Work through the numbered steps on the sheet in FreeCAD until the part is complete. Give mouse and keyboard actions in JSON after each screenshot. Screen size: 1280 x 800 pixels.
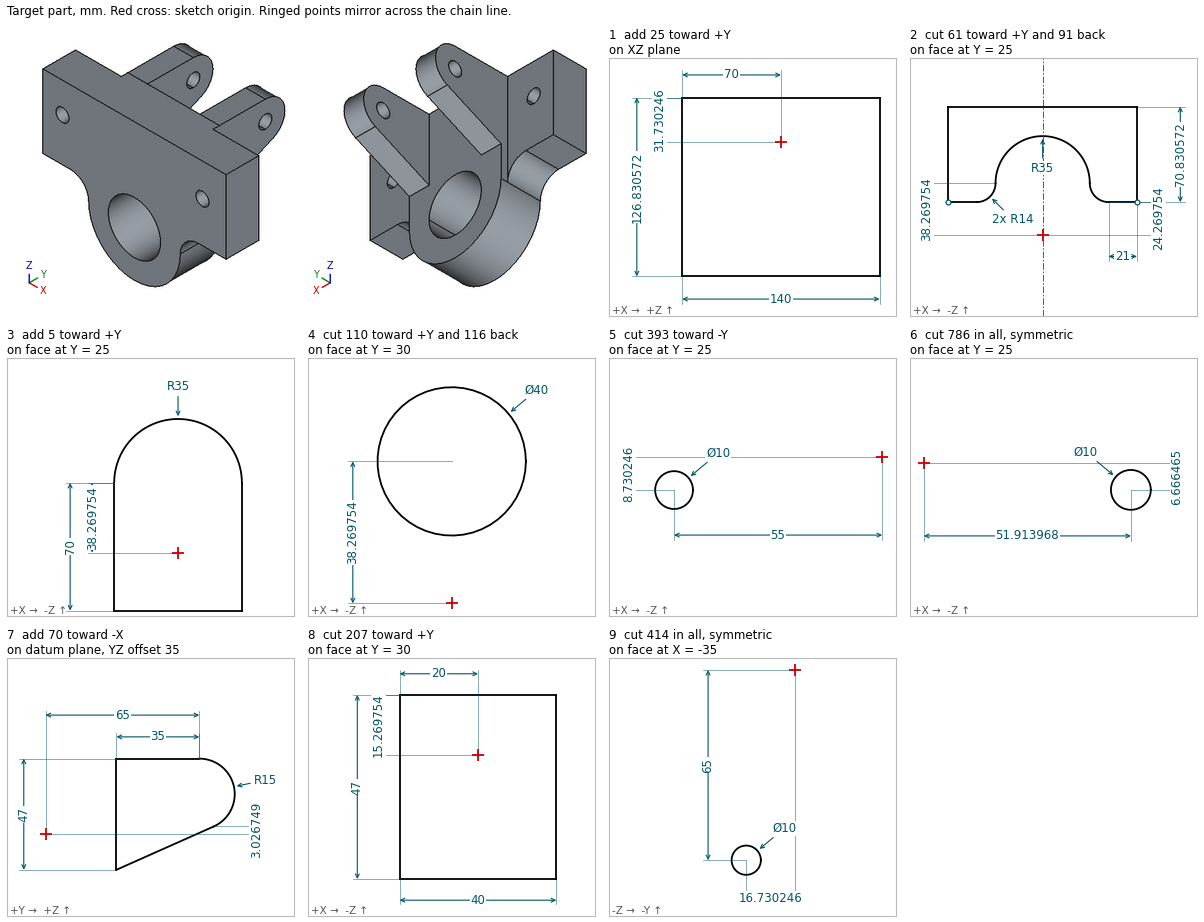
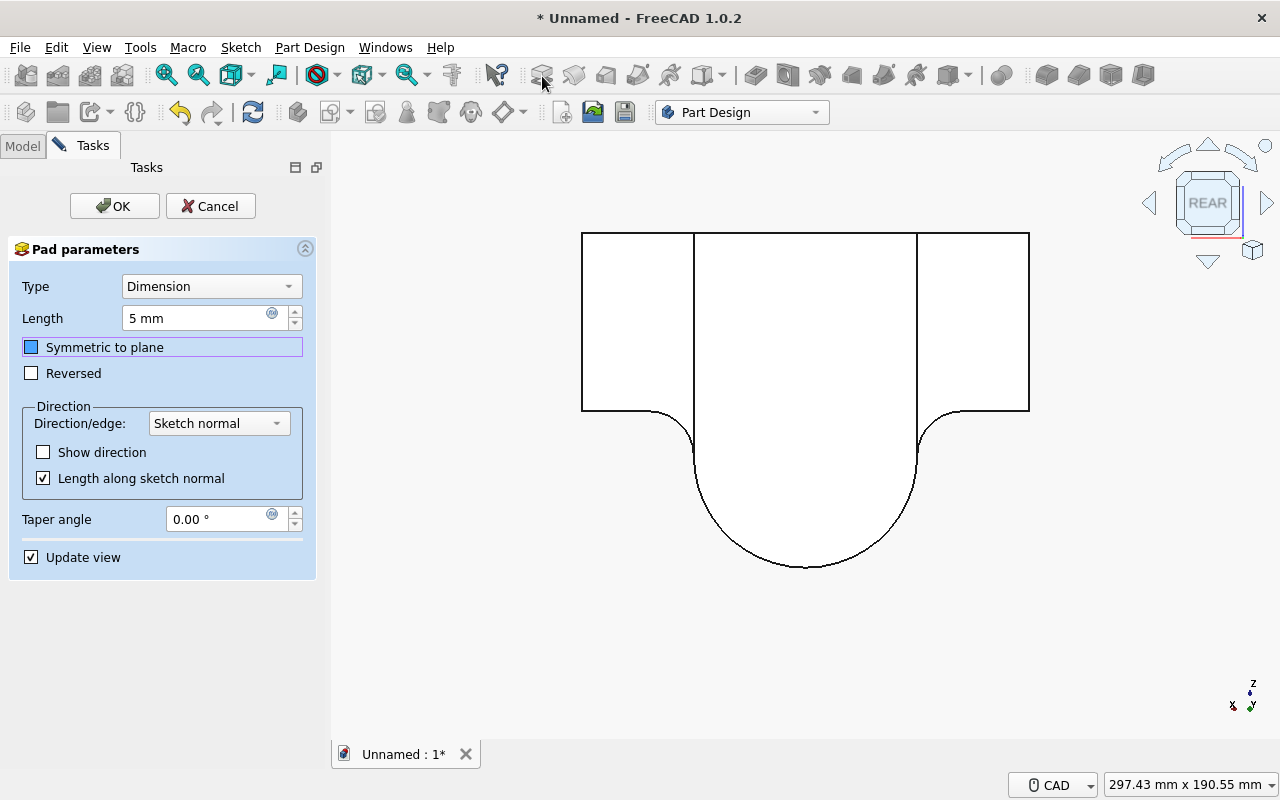
{"action": "left_click", "coordinate": [115, 206]}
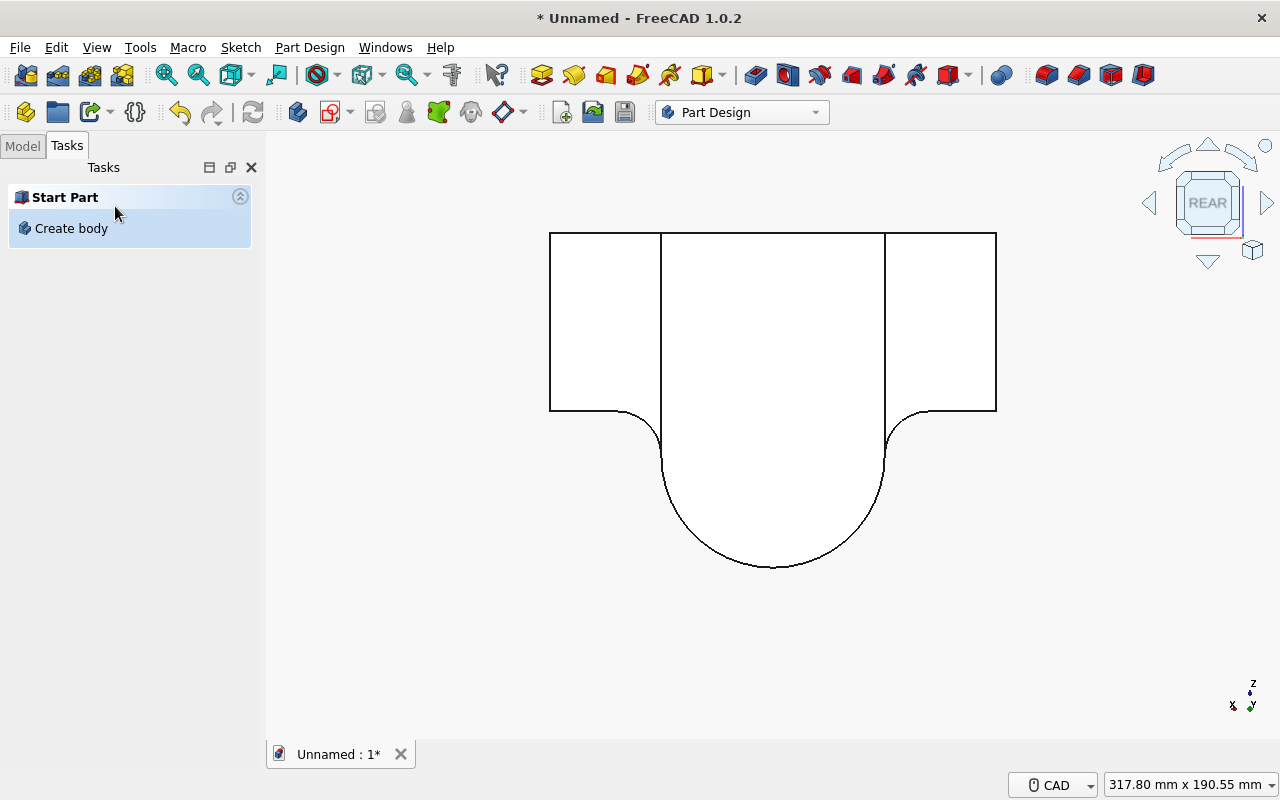
{"action": "left_click", "coordinate": [773, 351]}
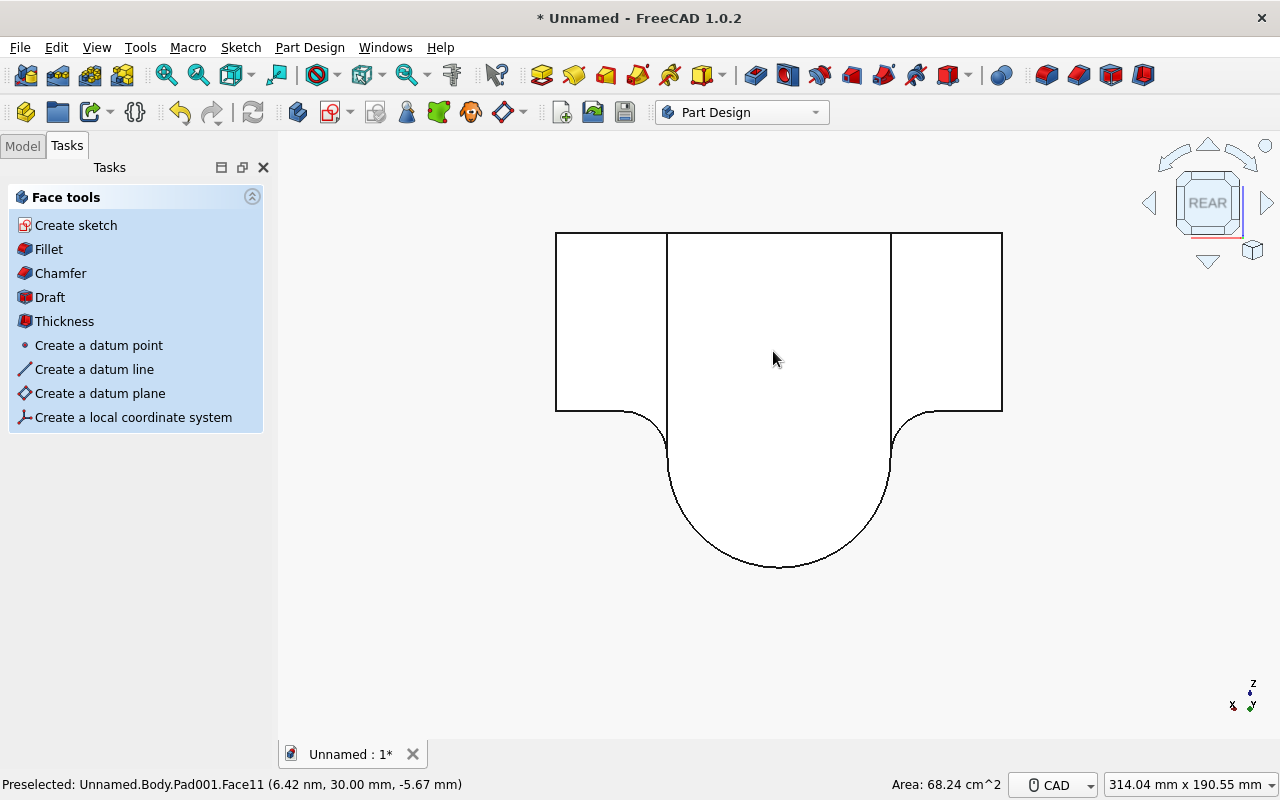
{"action": "left_click", "coordinate": [330, 112]}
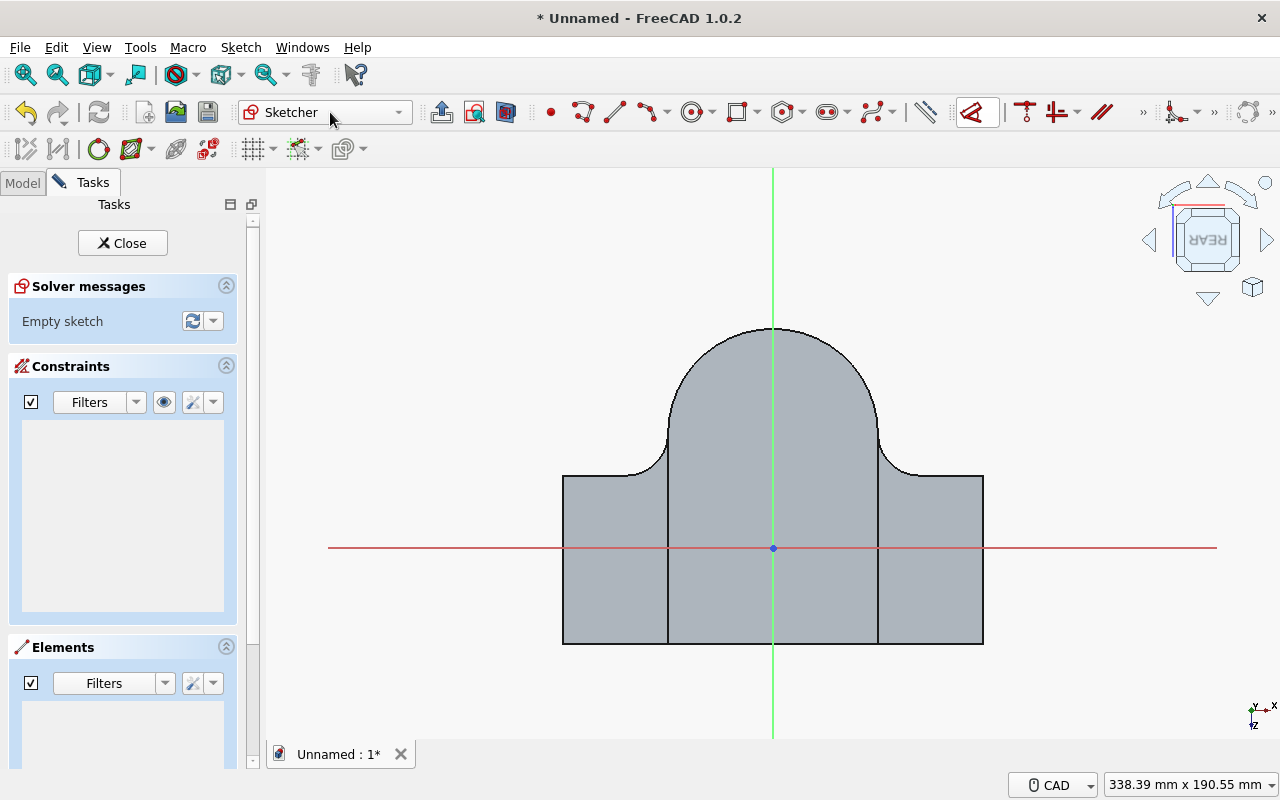
{"action": "scroll", "coordinate": [829, 467], "scroll_direction": "up", "scroll_amount": 4}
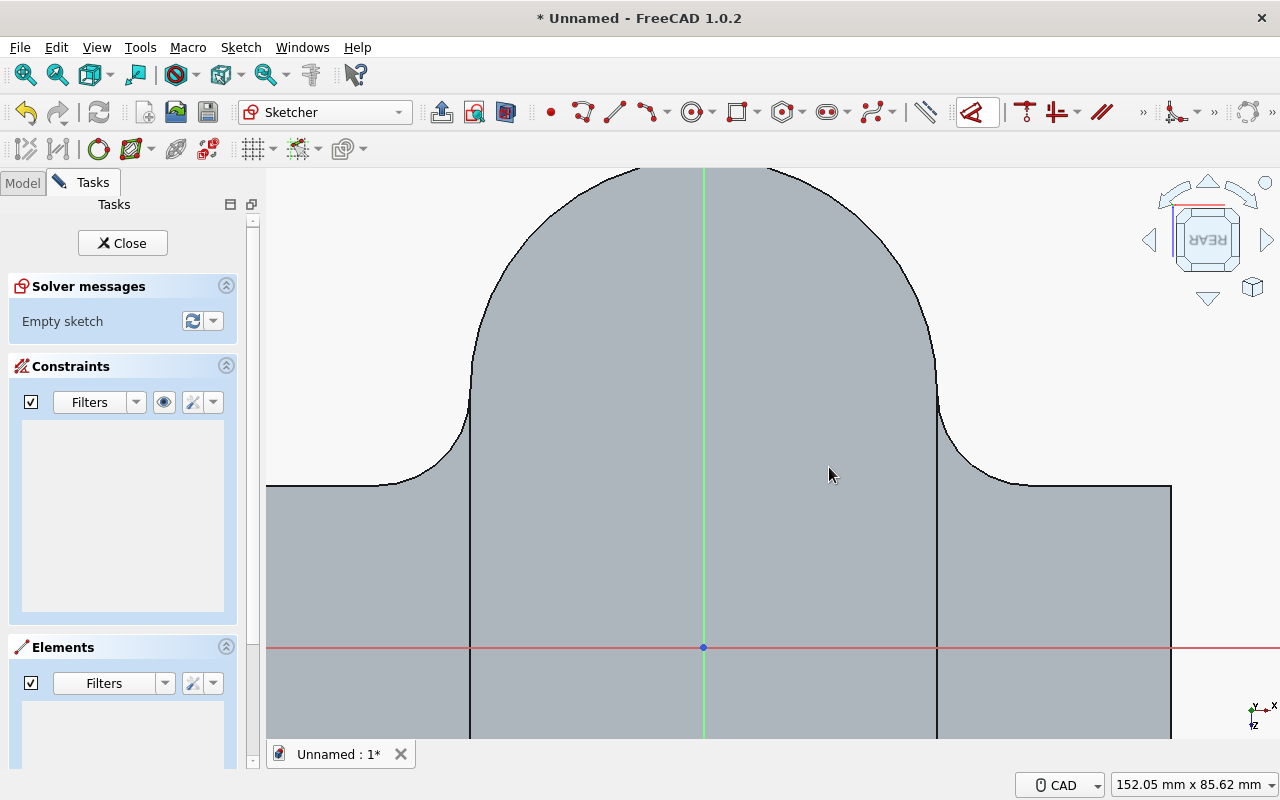
{"action": "left_click", "coordinate": [692, 112]}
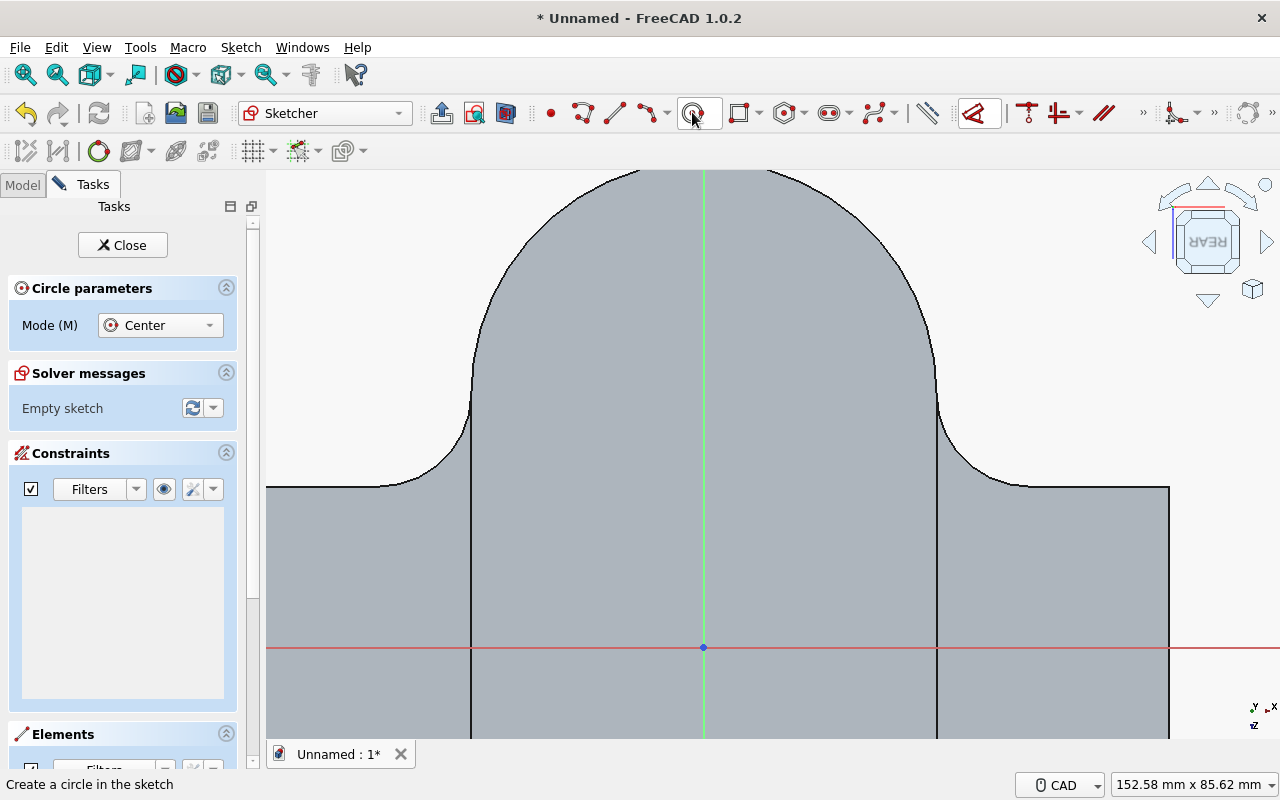
{"action": "left_click", "coordinate": [704, 394]}
{"action": "left_click", "coordinate": [798, 300]}
{"action": "key", "text": "Escape"}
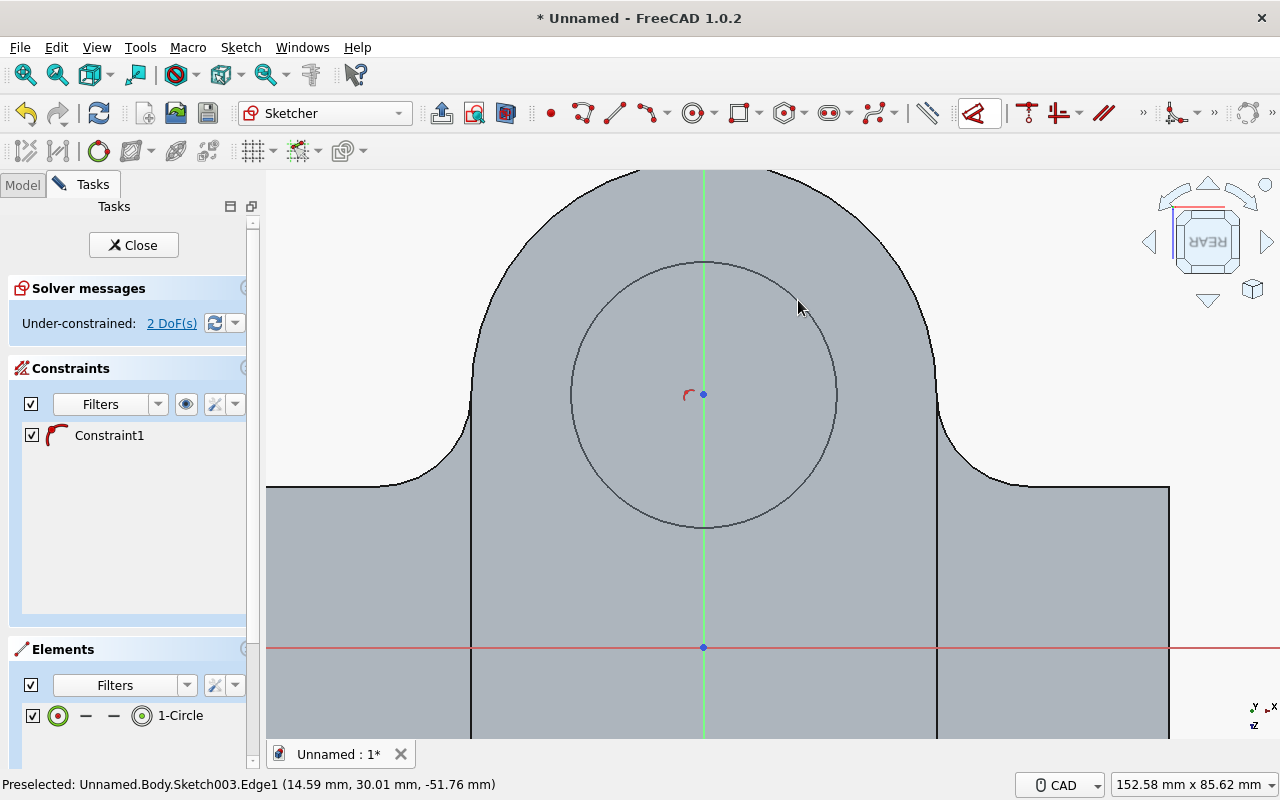
{"action": "left_click", "coordinate": [798, 301]}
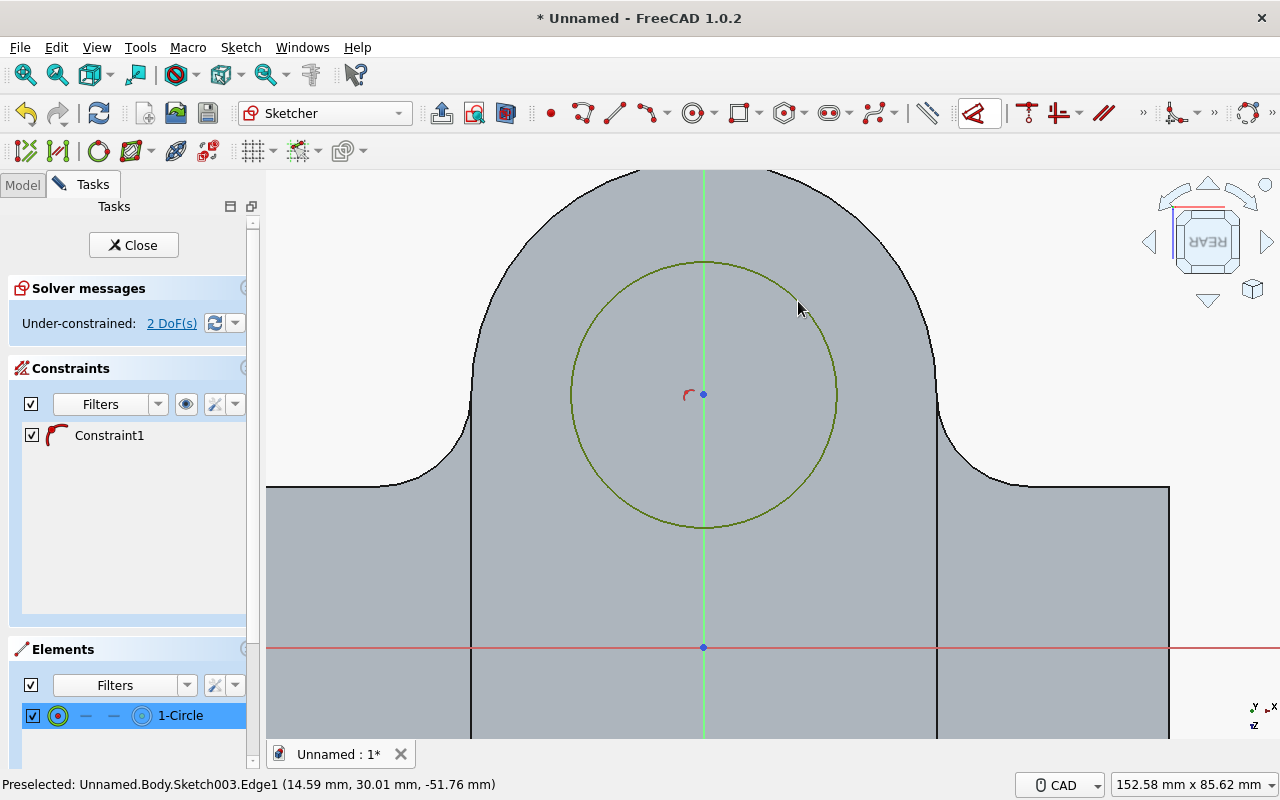
{"action": "left_click", "coordinate": [996, 114]}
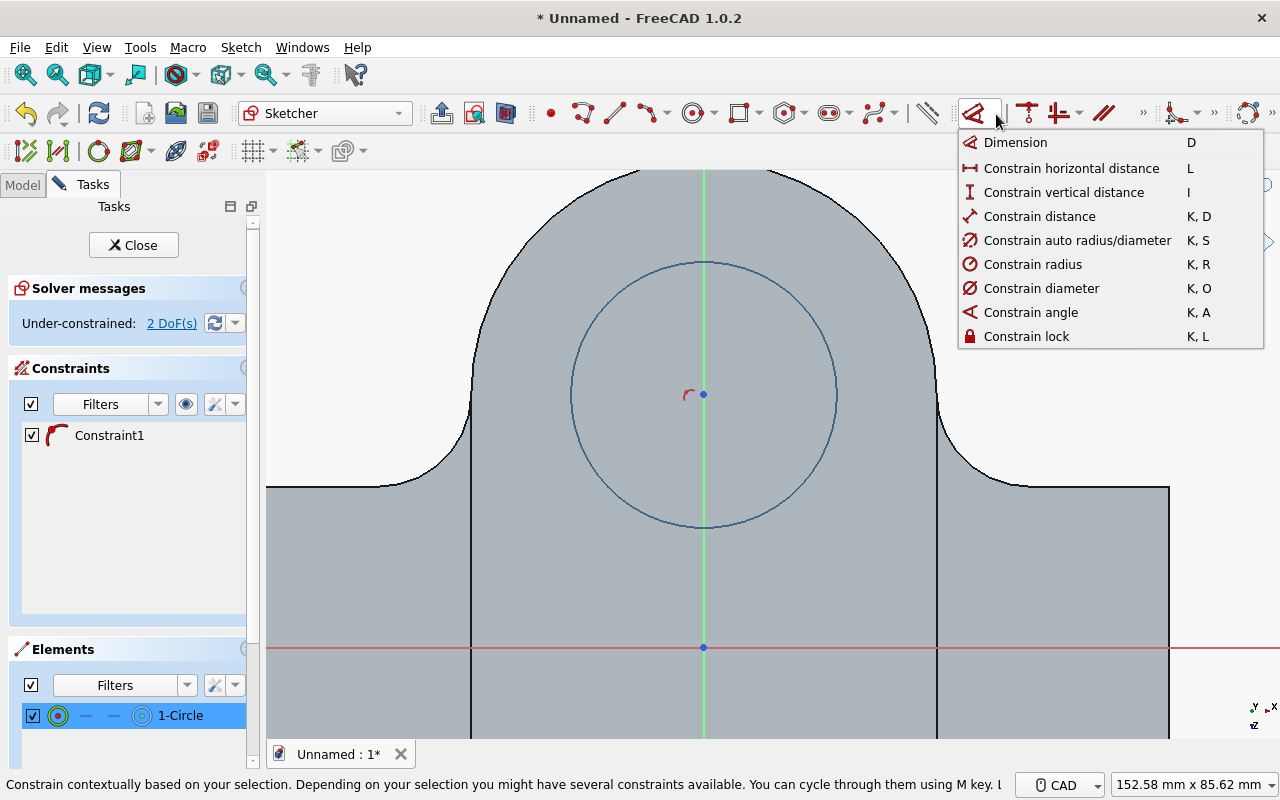
{"action": "left_click", "coordinate": [1111, 288]}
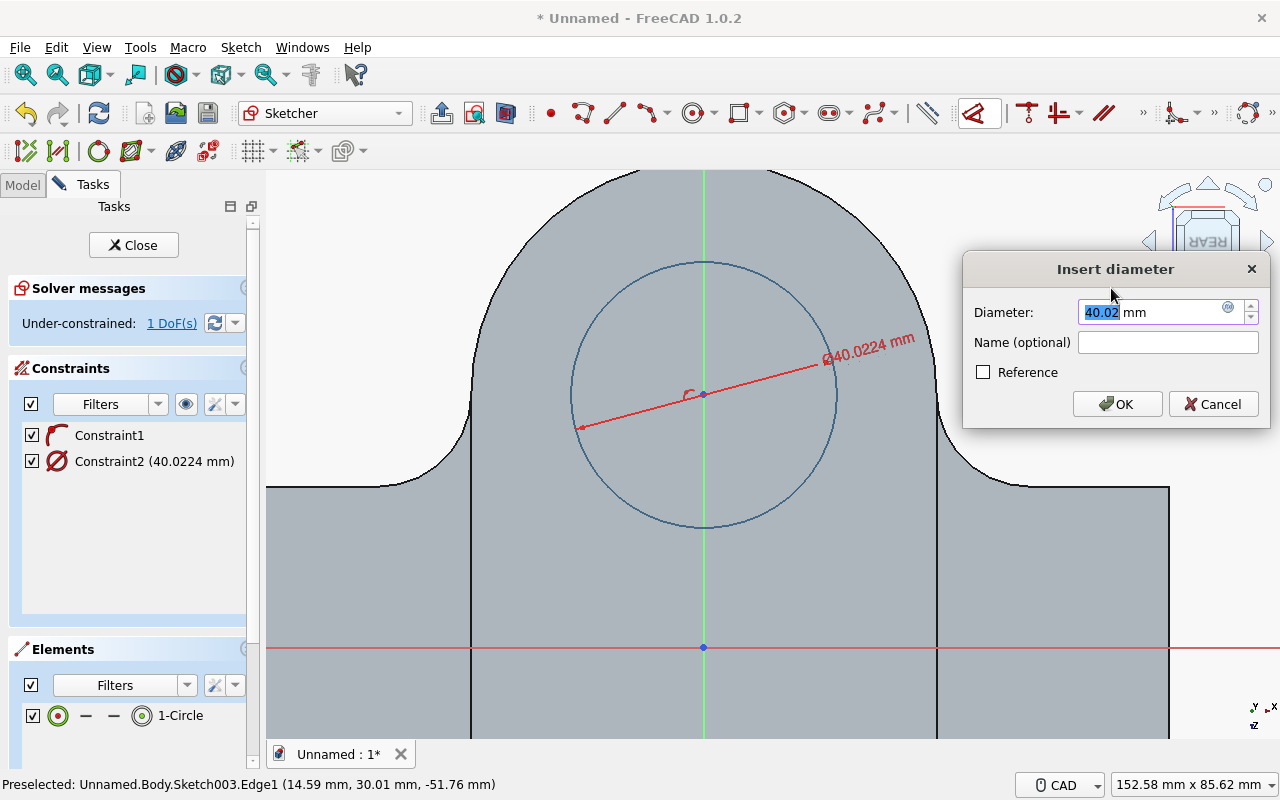
{"action": "type", "text": "40"}
{"action": "key", "text": "Return"}